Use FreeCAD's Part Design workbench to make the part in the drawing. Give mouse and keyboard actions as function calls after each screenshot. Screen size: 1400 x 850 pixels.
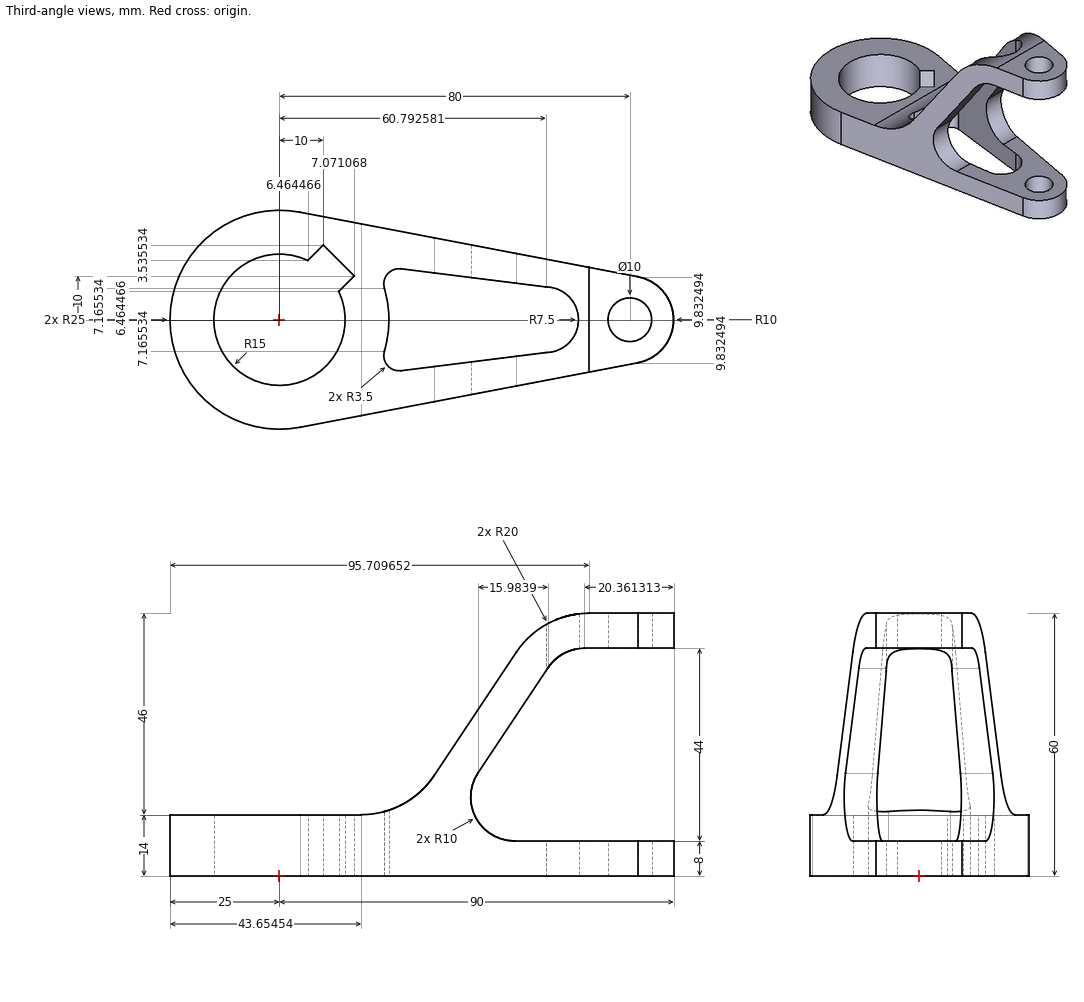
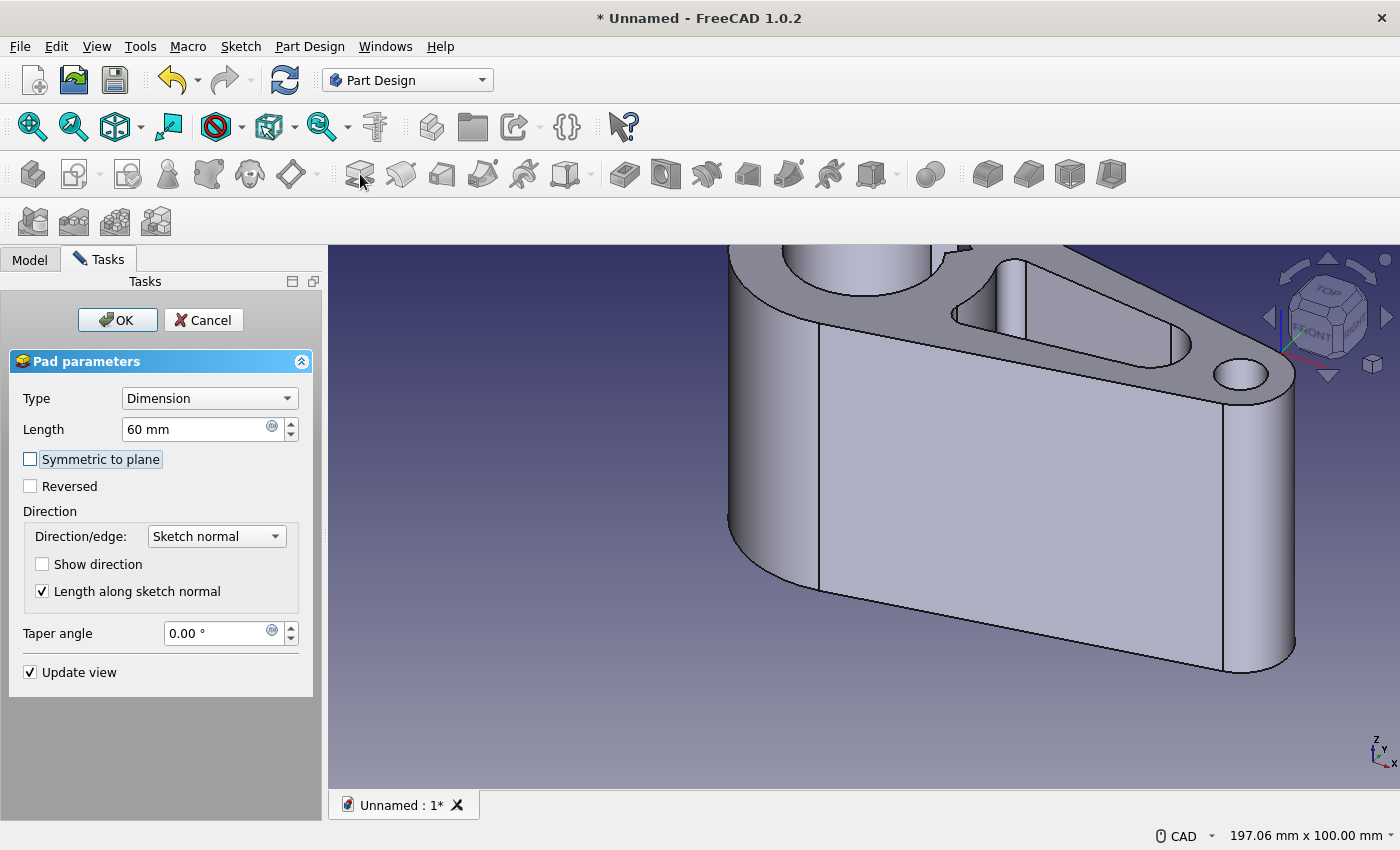
click(118, 320)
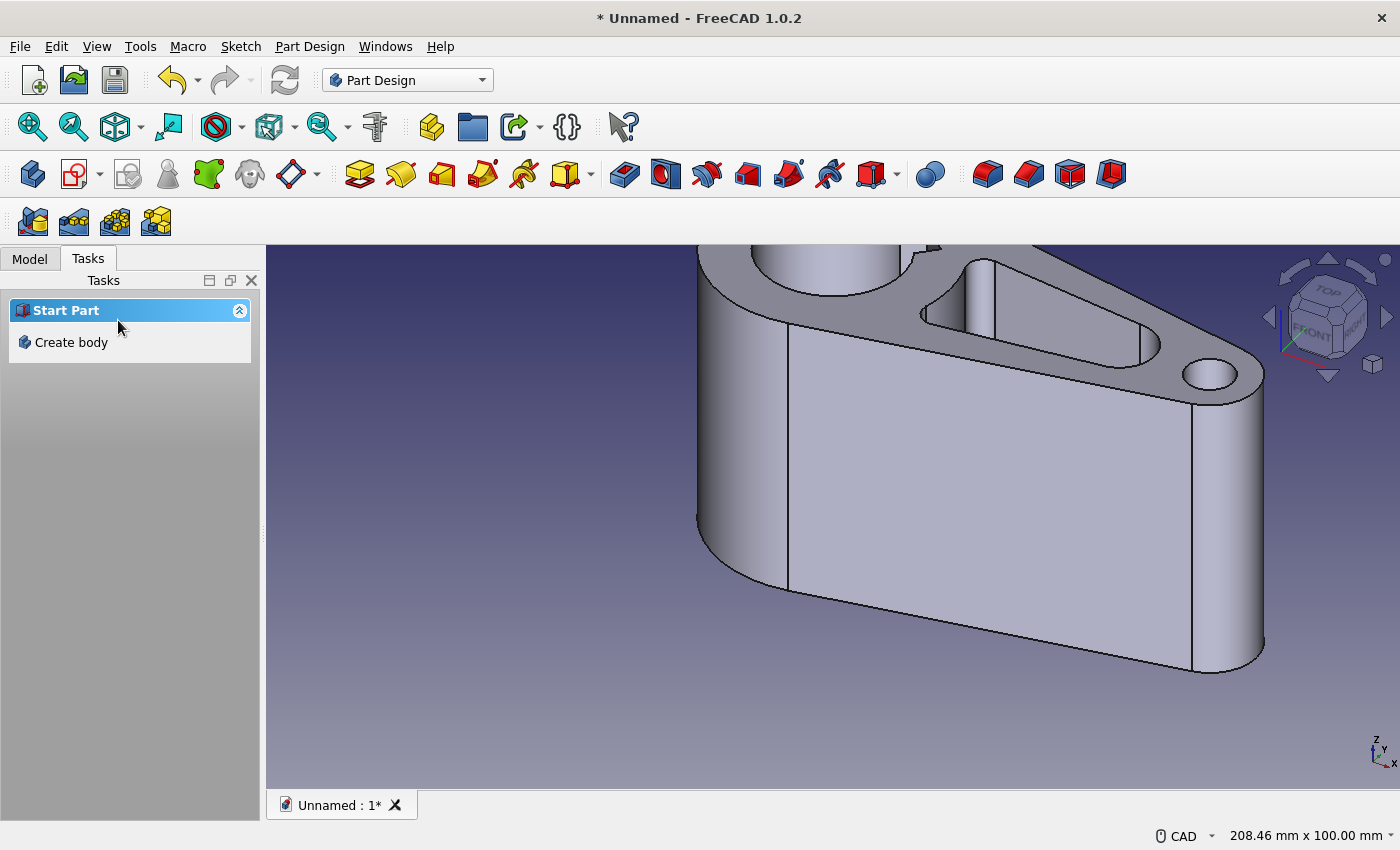
click(33, 128)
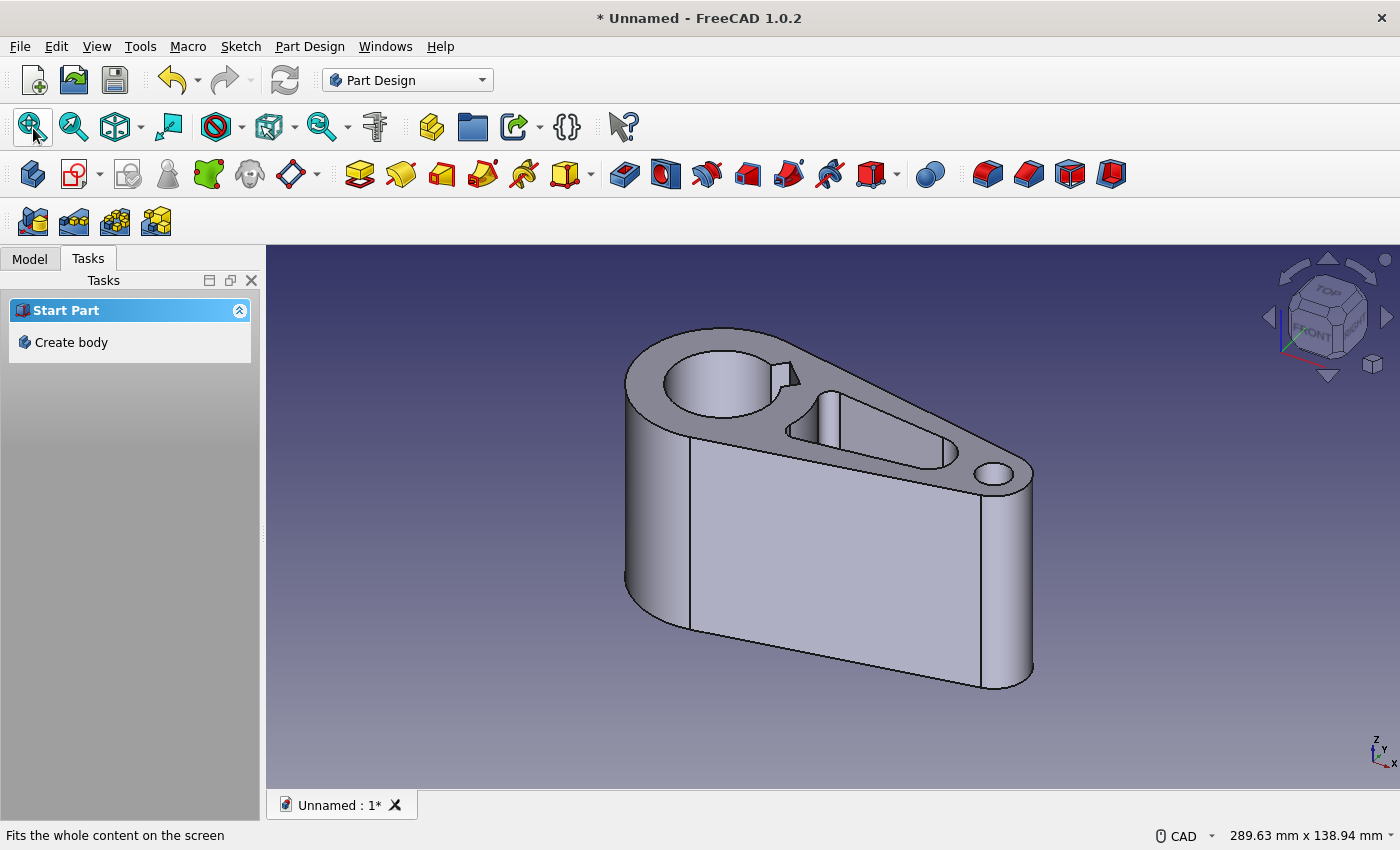
click(74, 174)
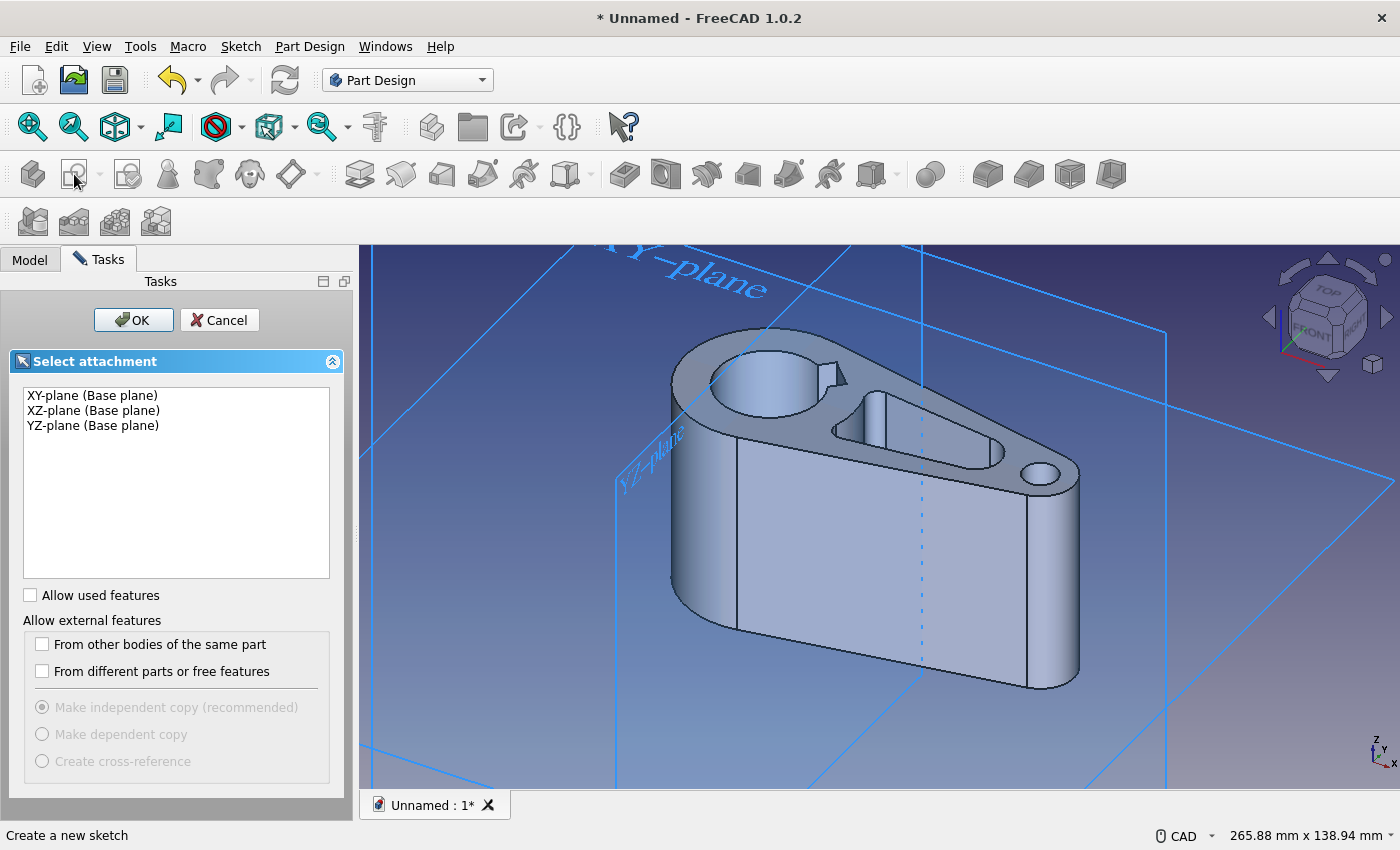
click(84, 410)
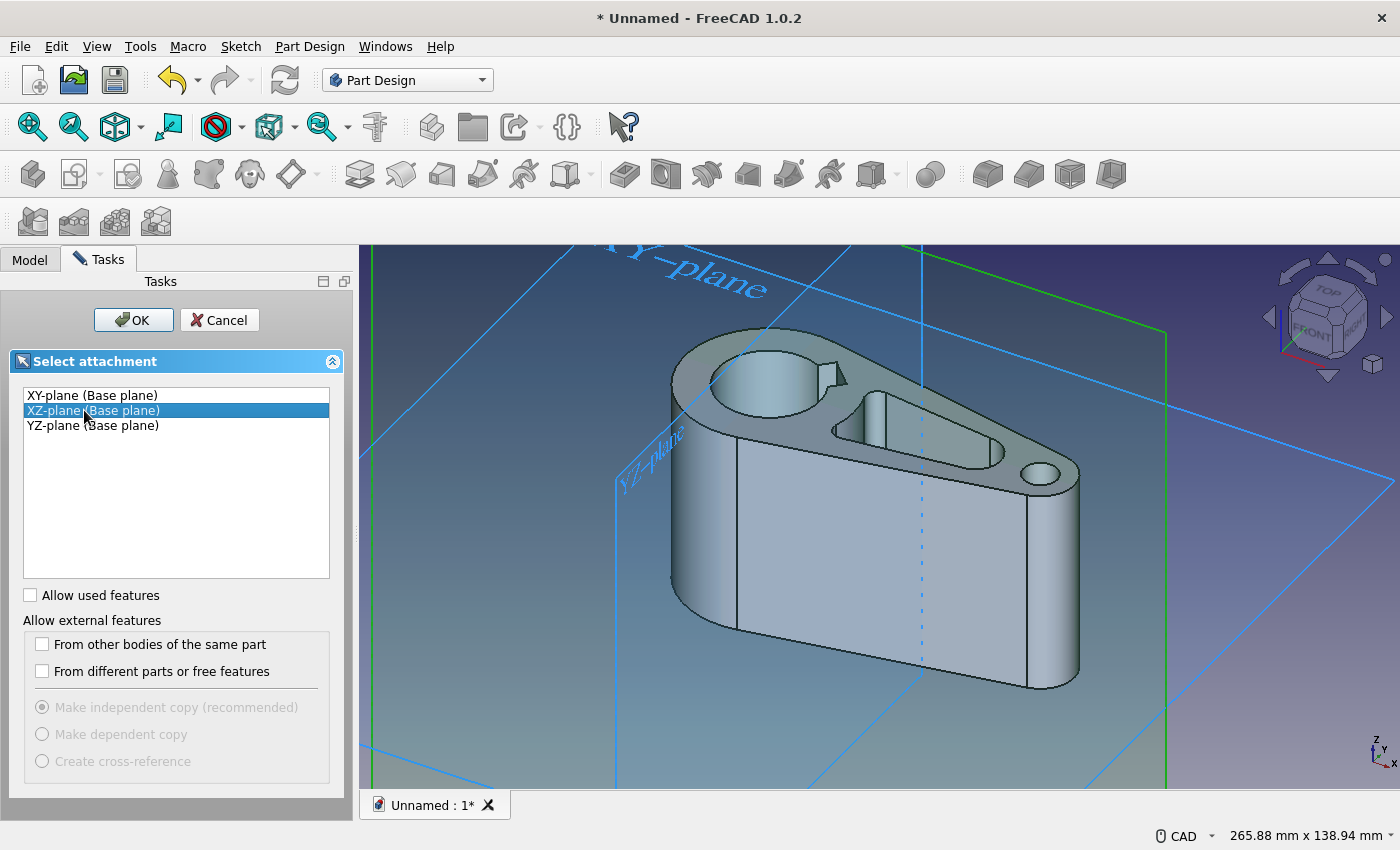
click(134, 320)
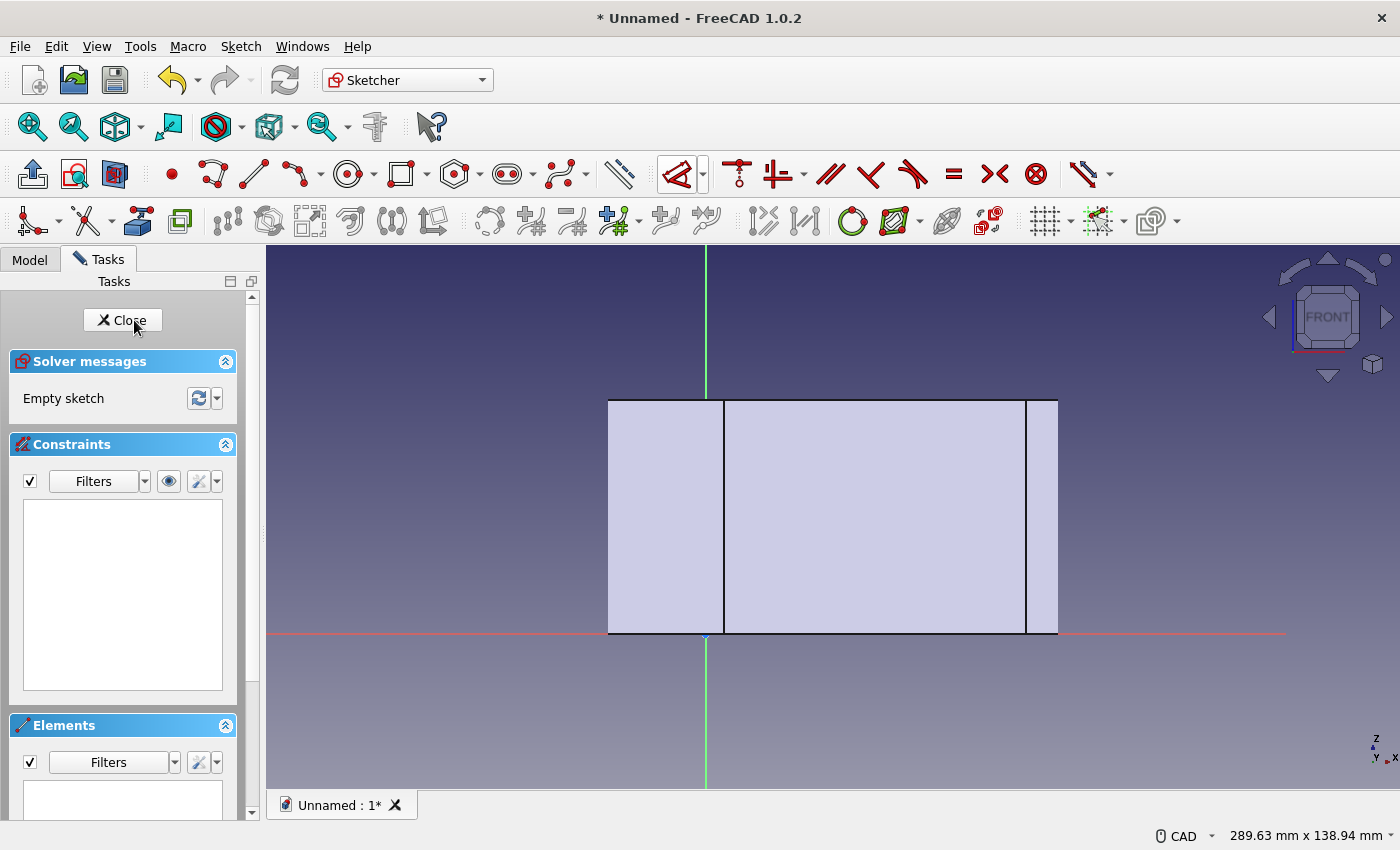
click(115, 174)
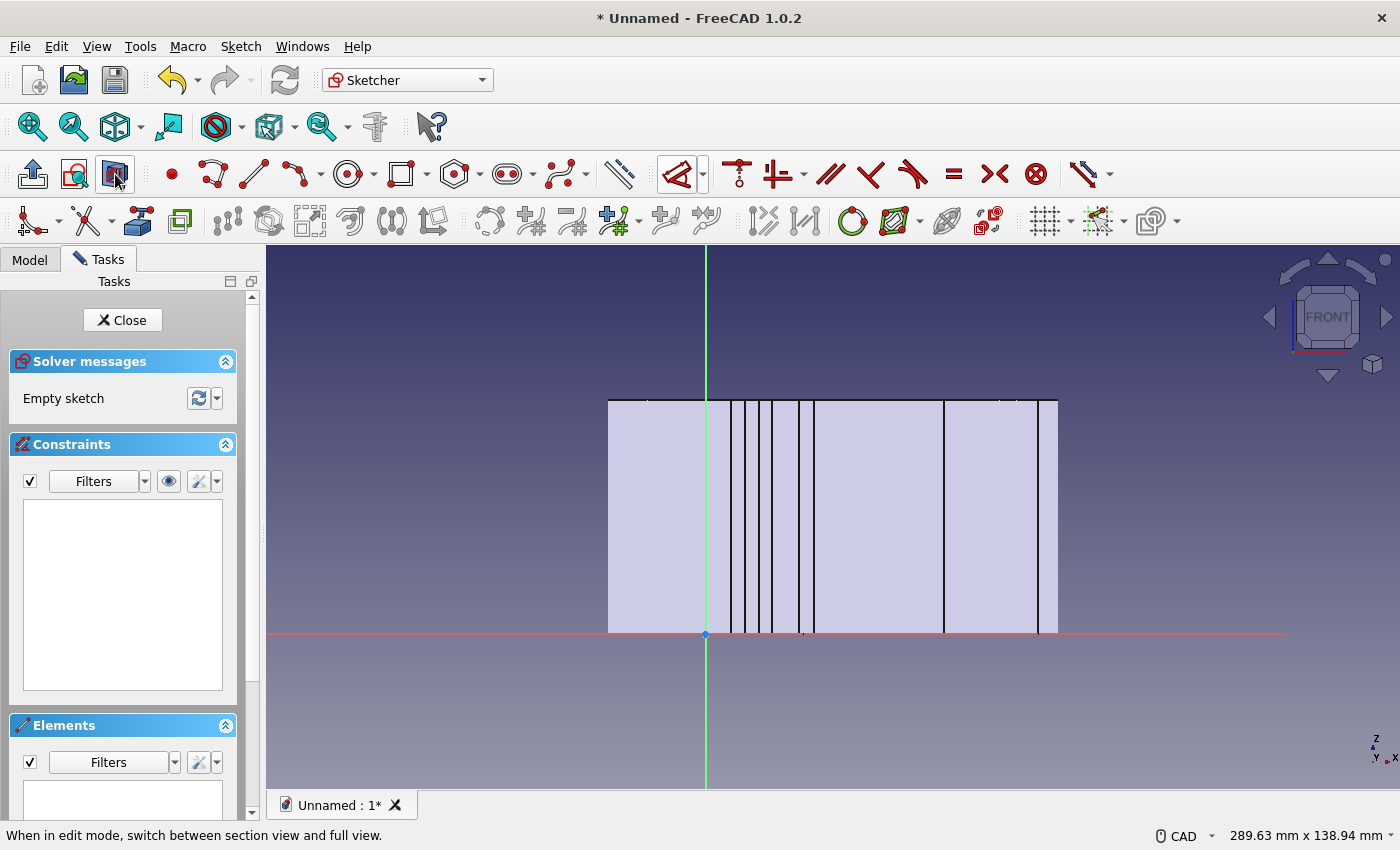
scroll(972, 517, up, 2)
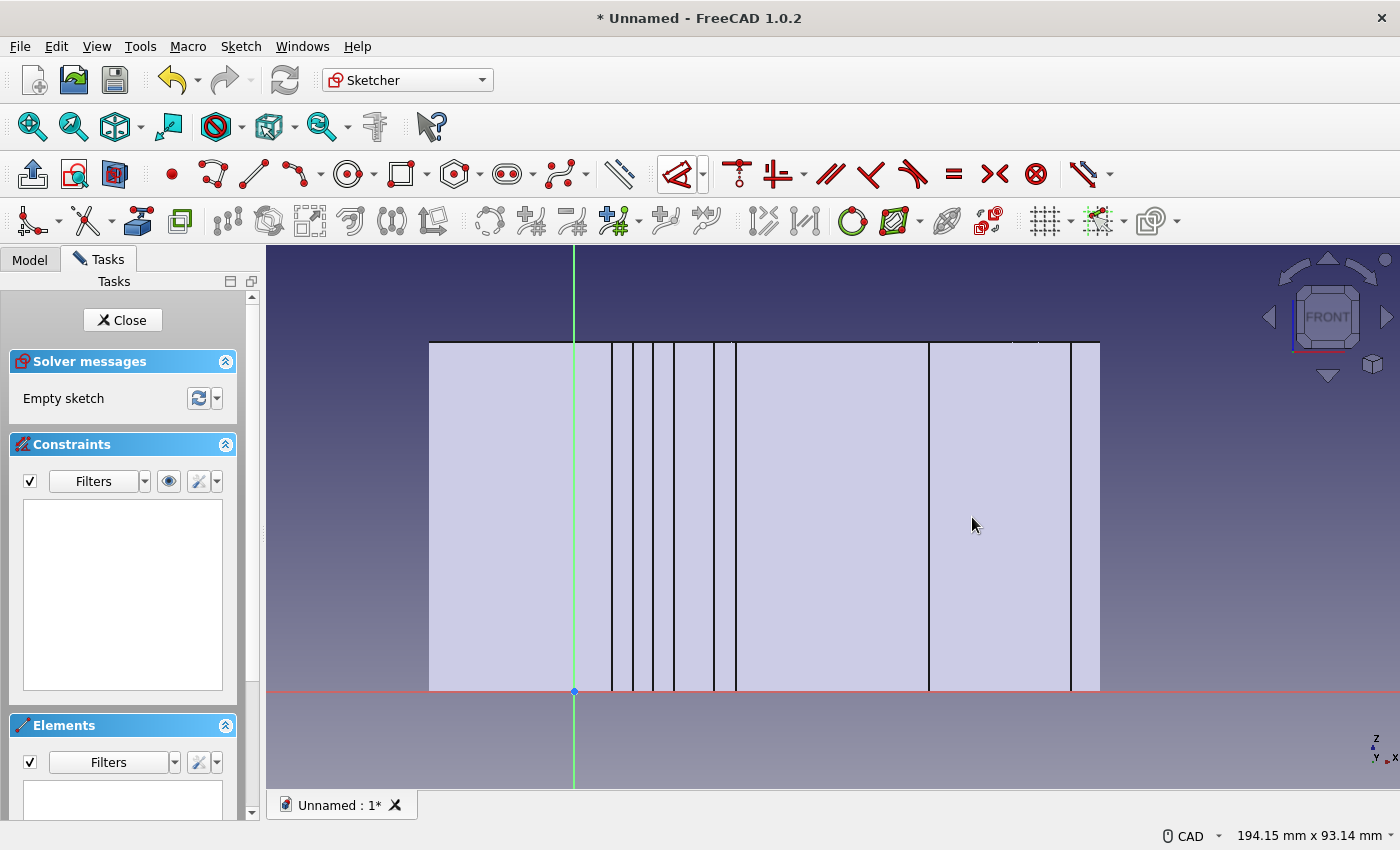
click(213, 174)